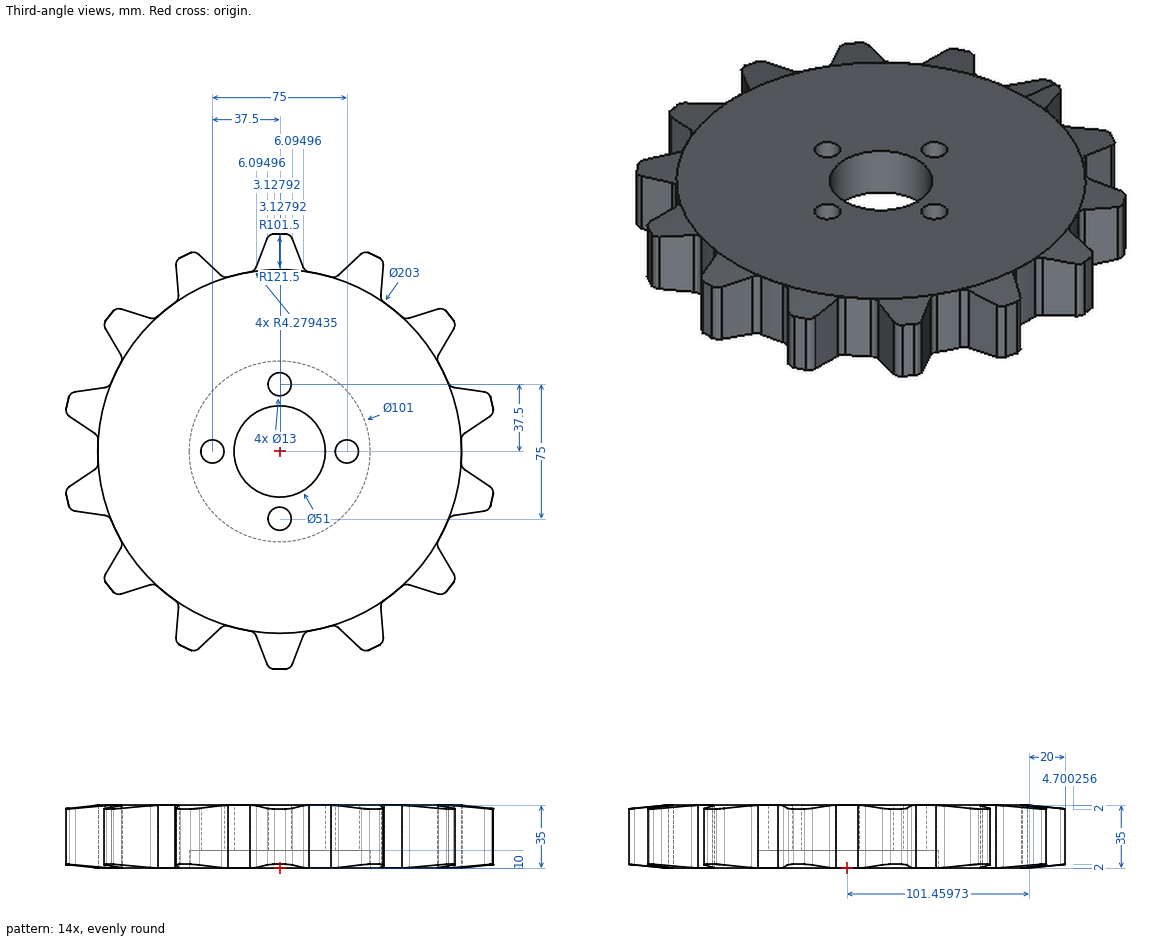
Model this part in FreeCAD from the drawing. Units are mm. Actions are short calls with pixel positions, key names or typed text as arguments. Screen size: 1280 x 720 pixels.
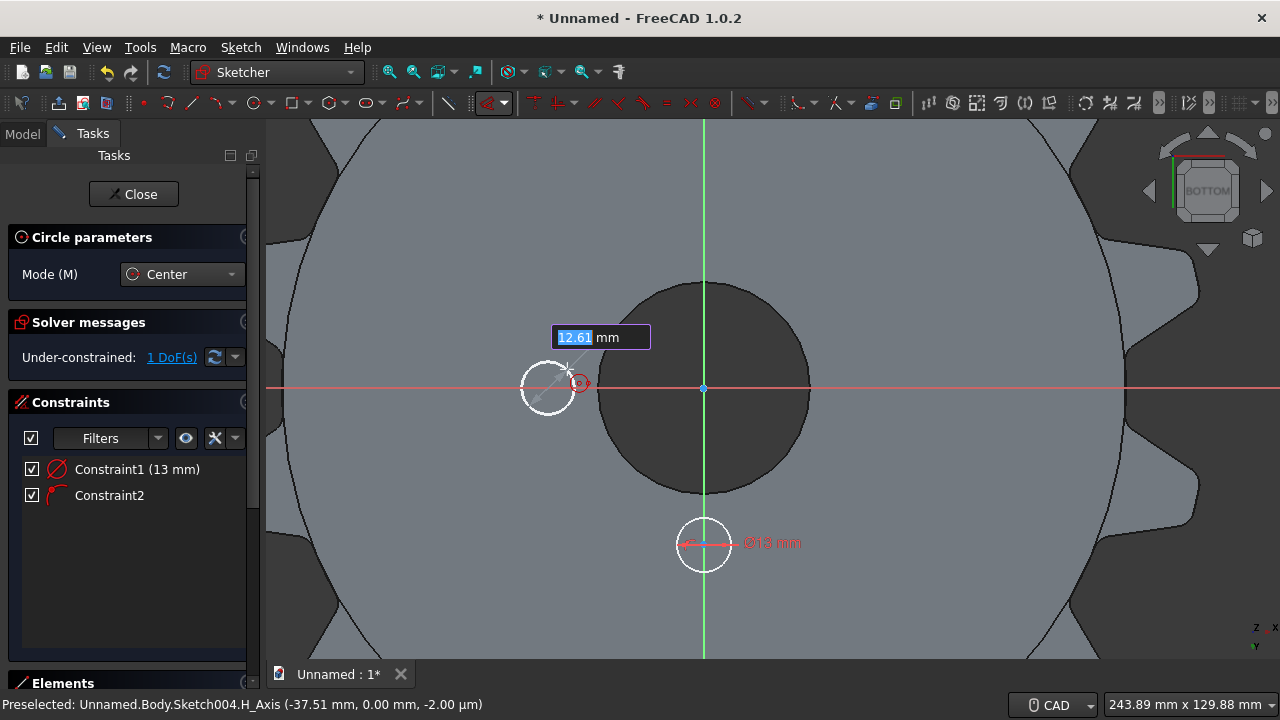
text(13)
key(Return)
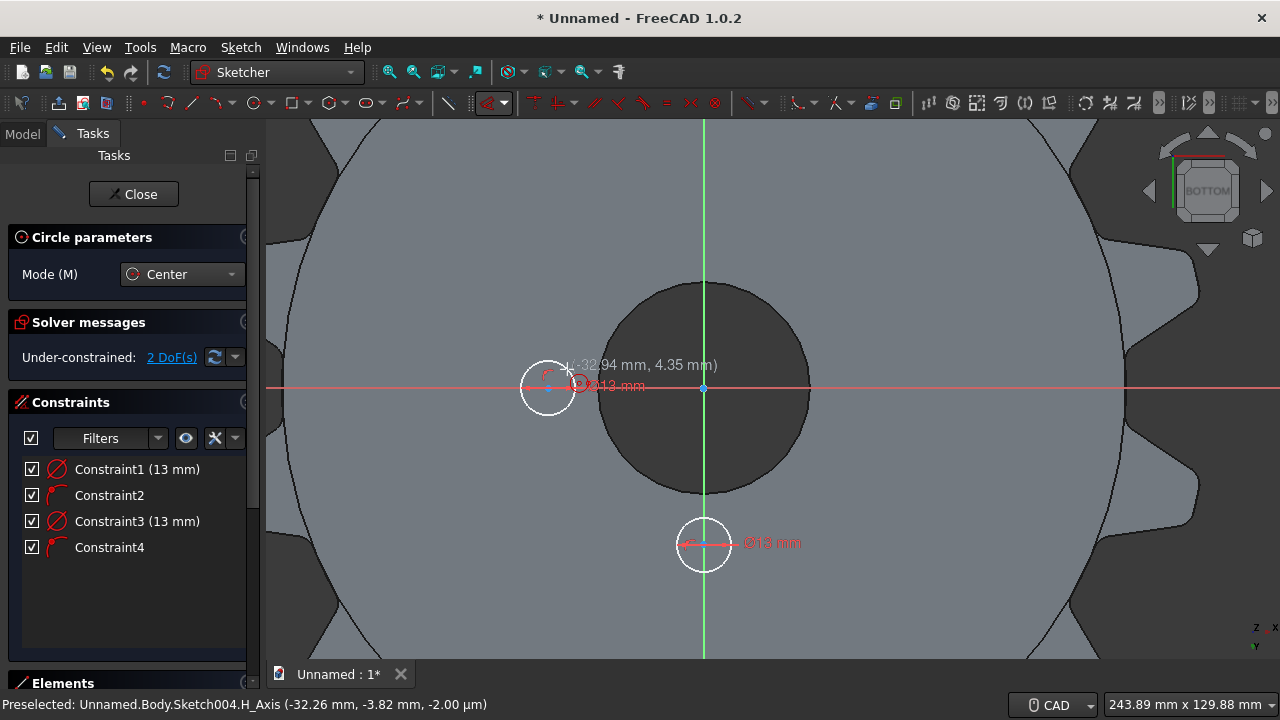
click(704, 232)
move(723, 213)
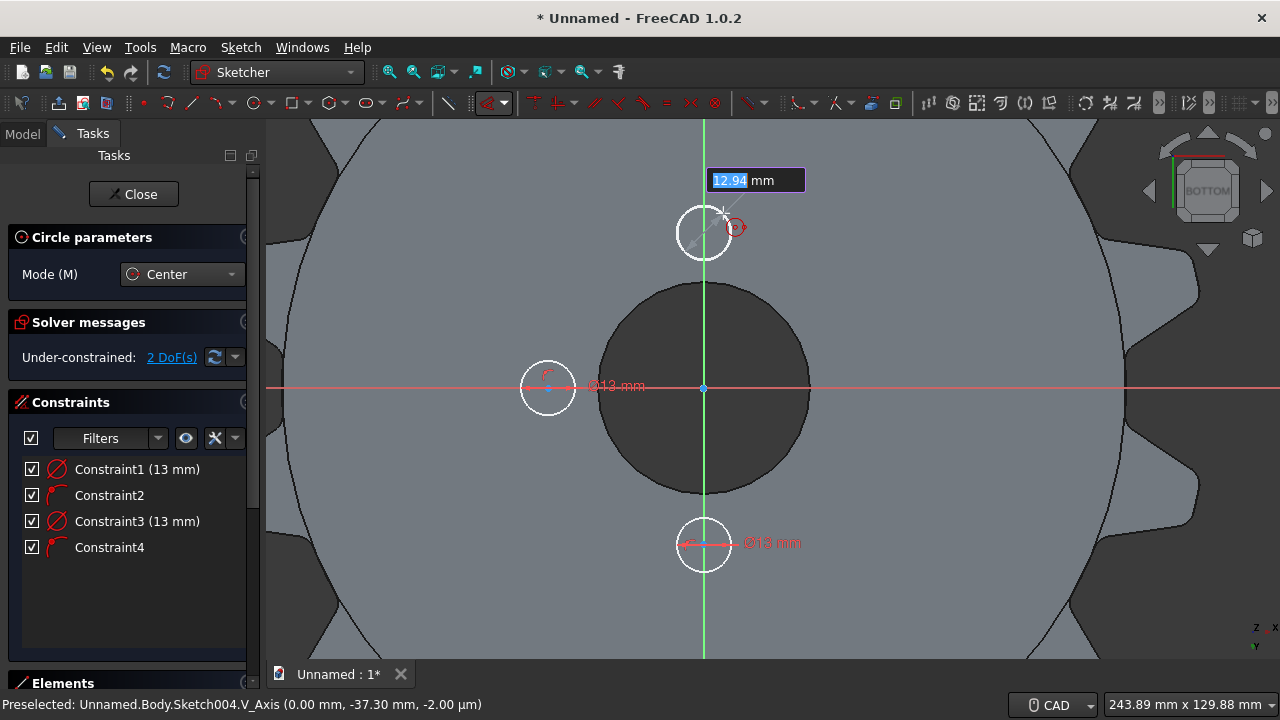
text(13)
key(Return)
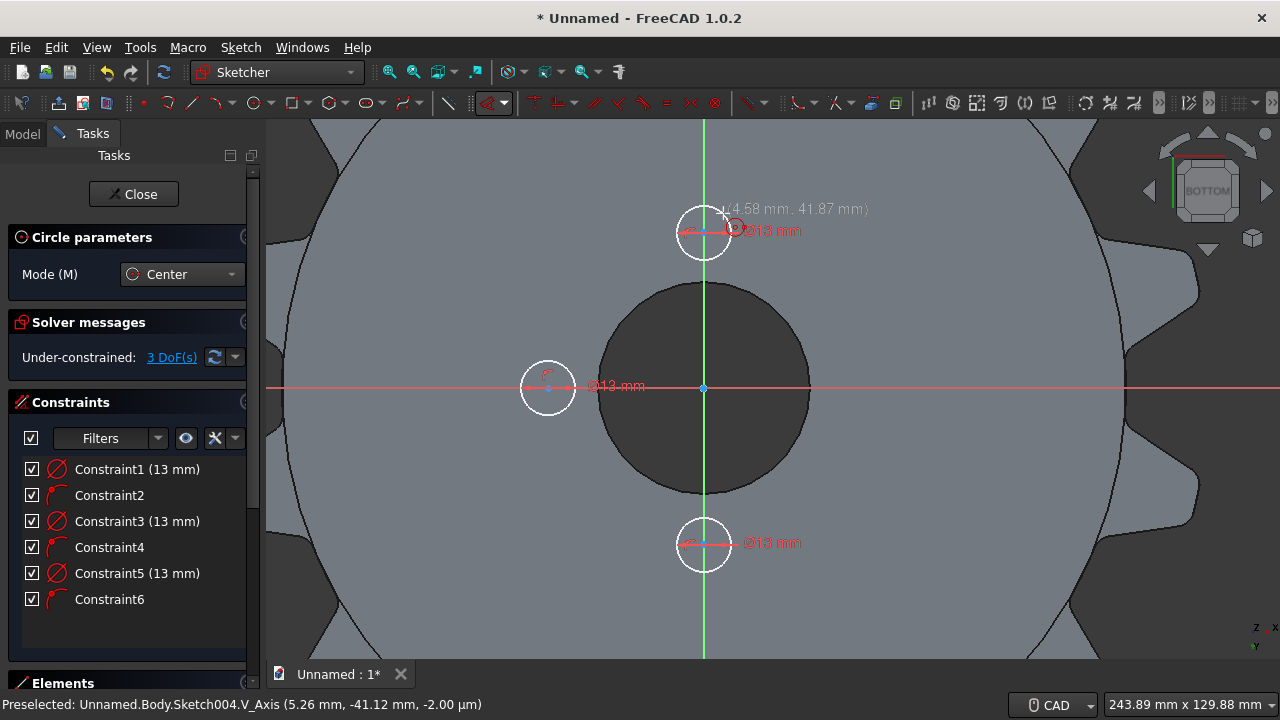
click(860, 388)
move(879, 369)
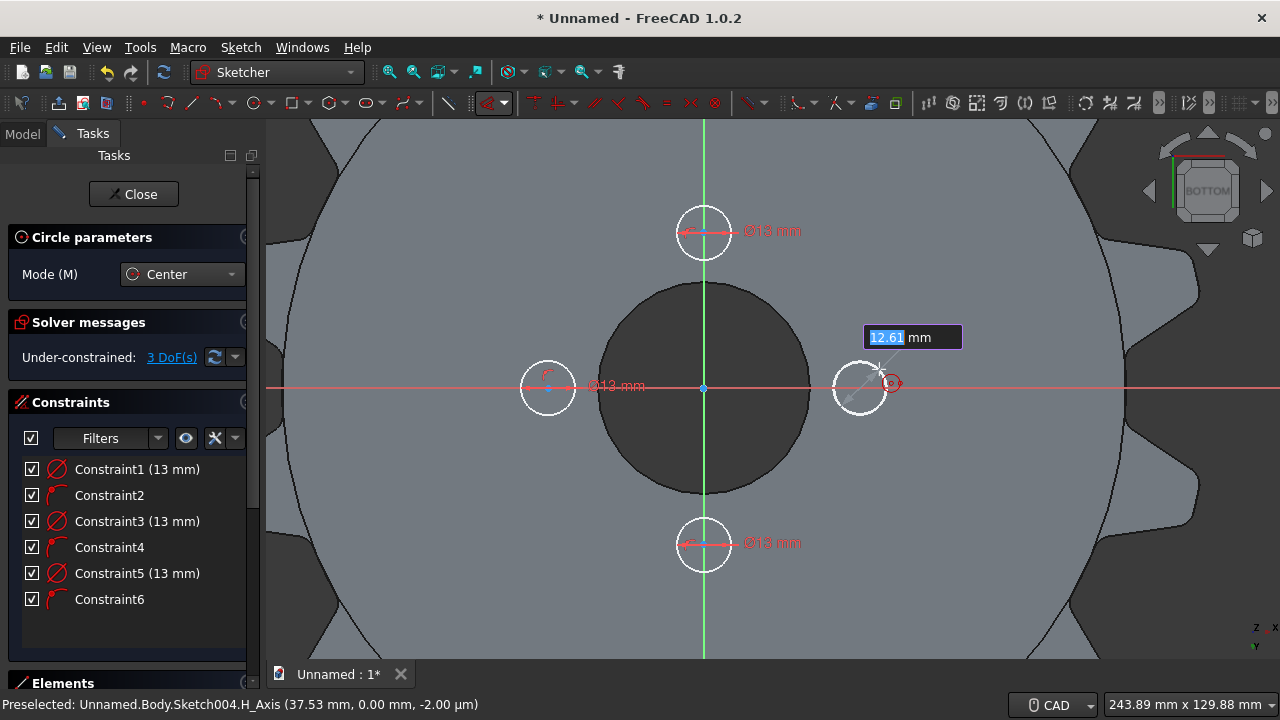
text(13)
key(Return)
key(Escape)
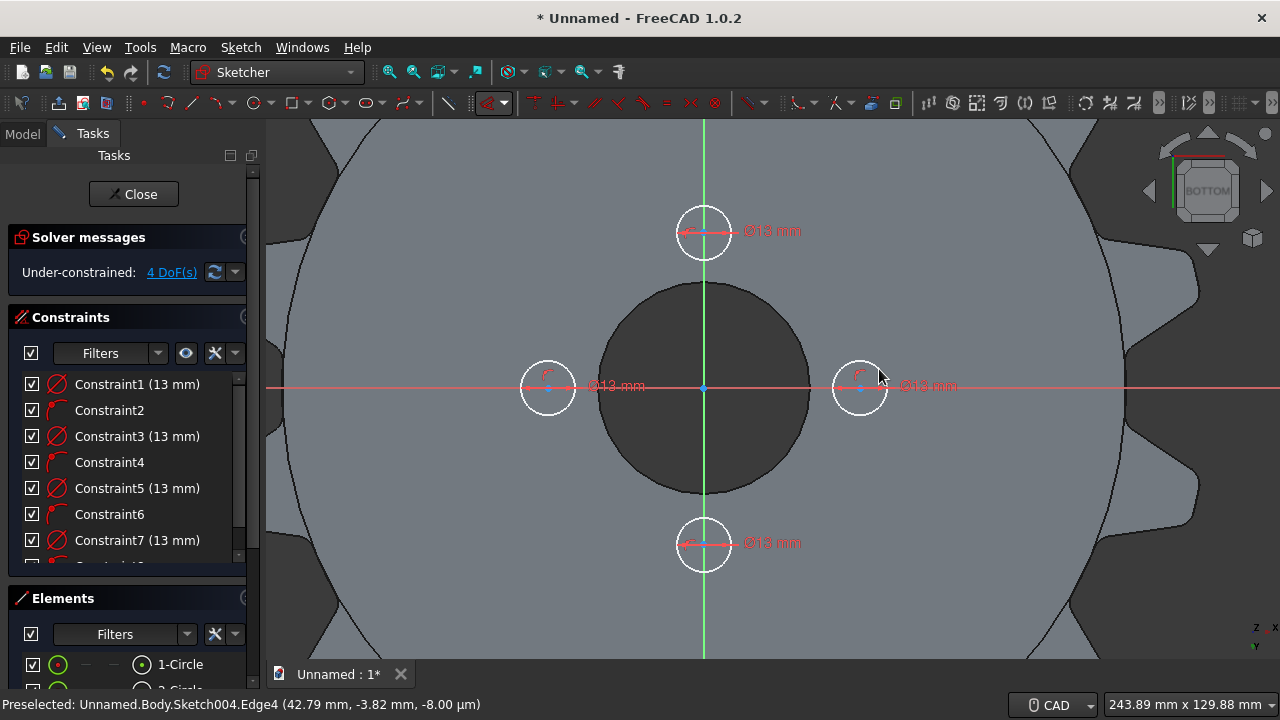
click(704, 545)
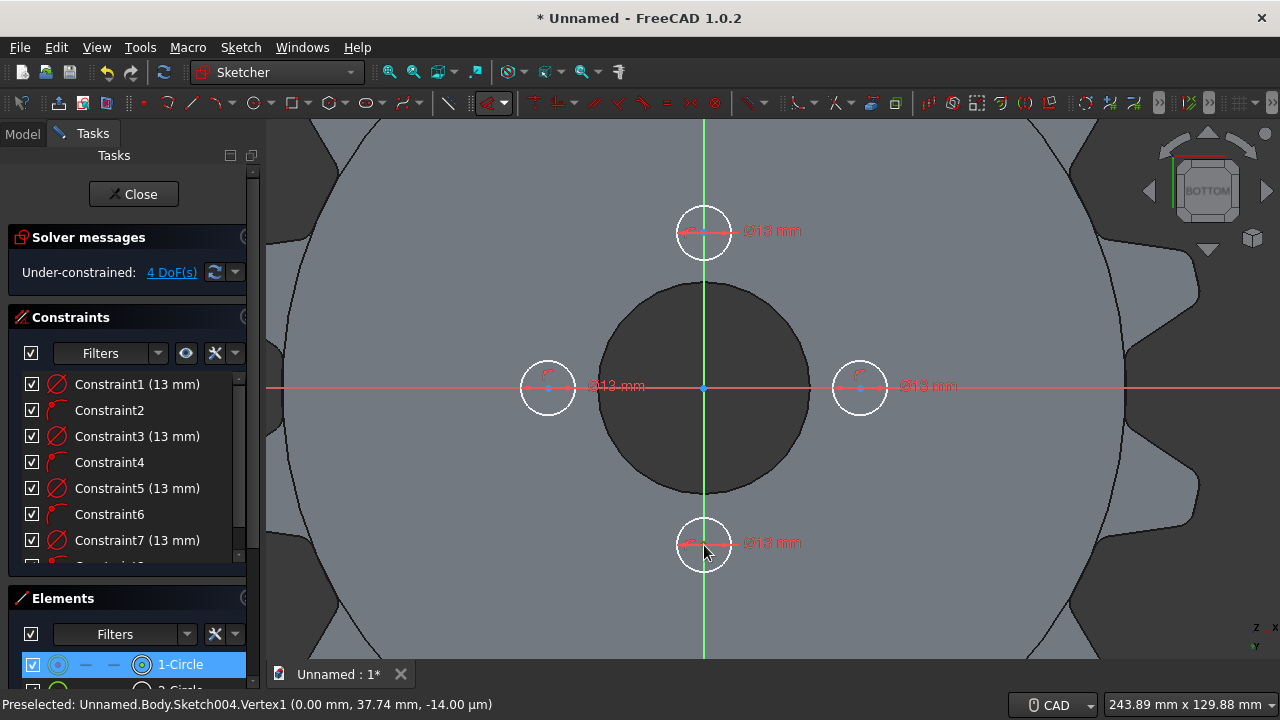
click(704, 233)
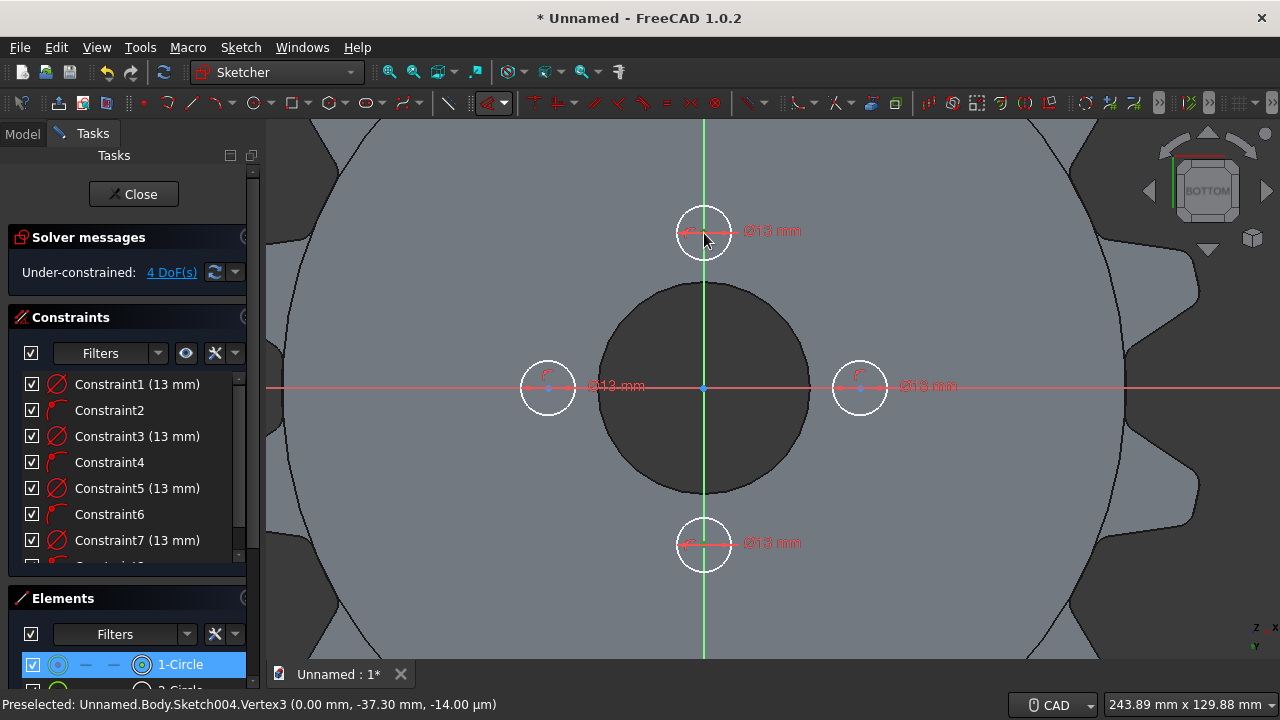
key(i)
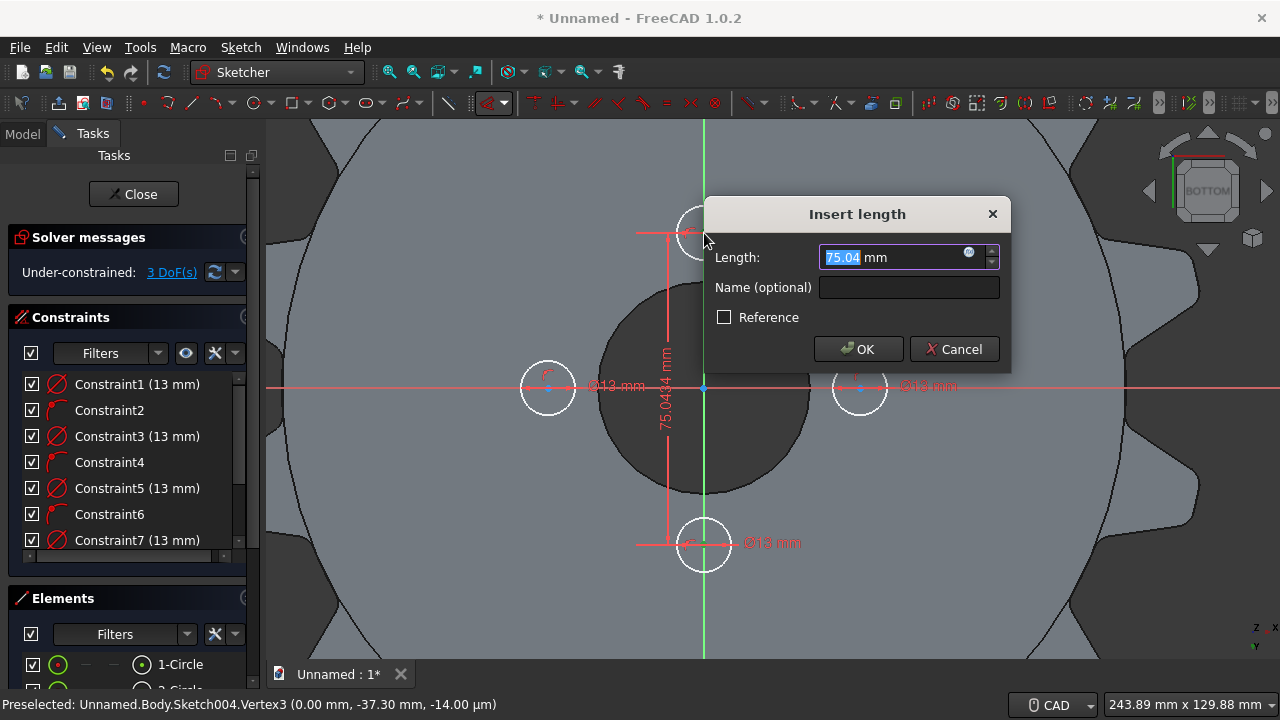
text(75)
key(Return)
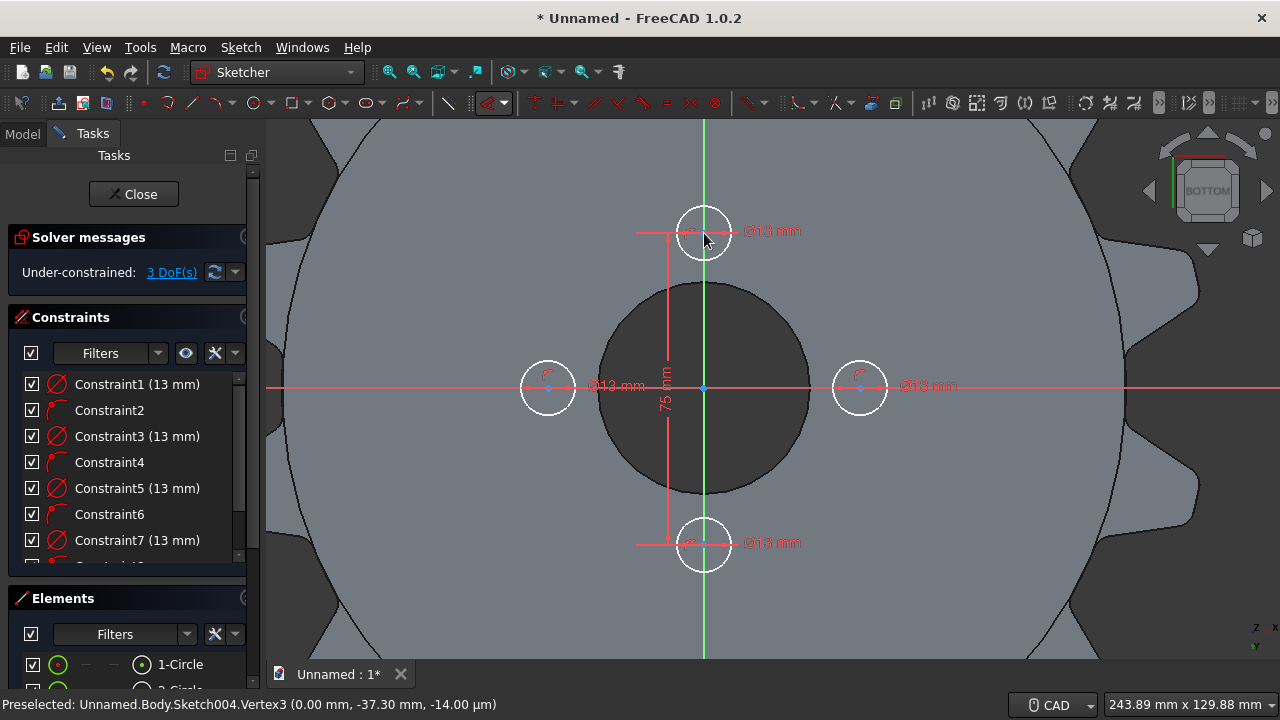
click(548, 388)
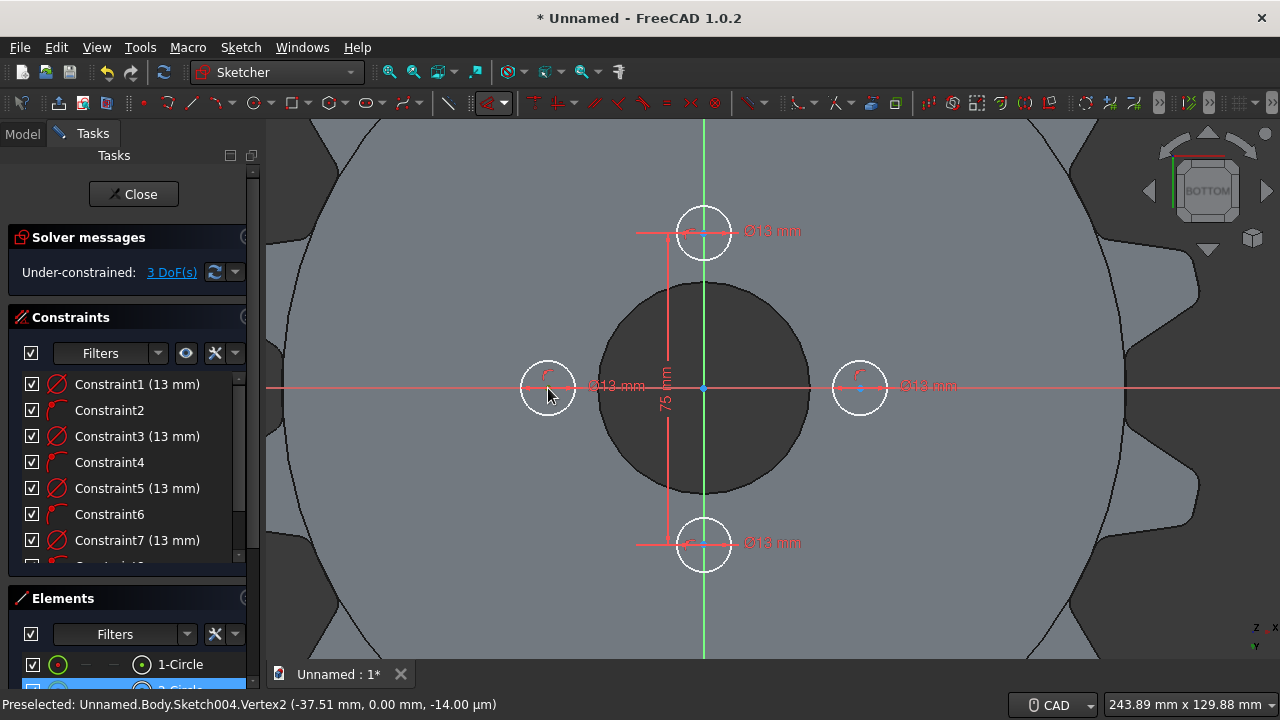
click(860, 388)